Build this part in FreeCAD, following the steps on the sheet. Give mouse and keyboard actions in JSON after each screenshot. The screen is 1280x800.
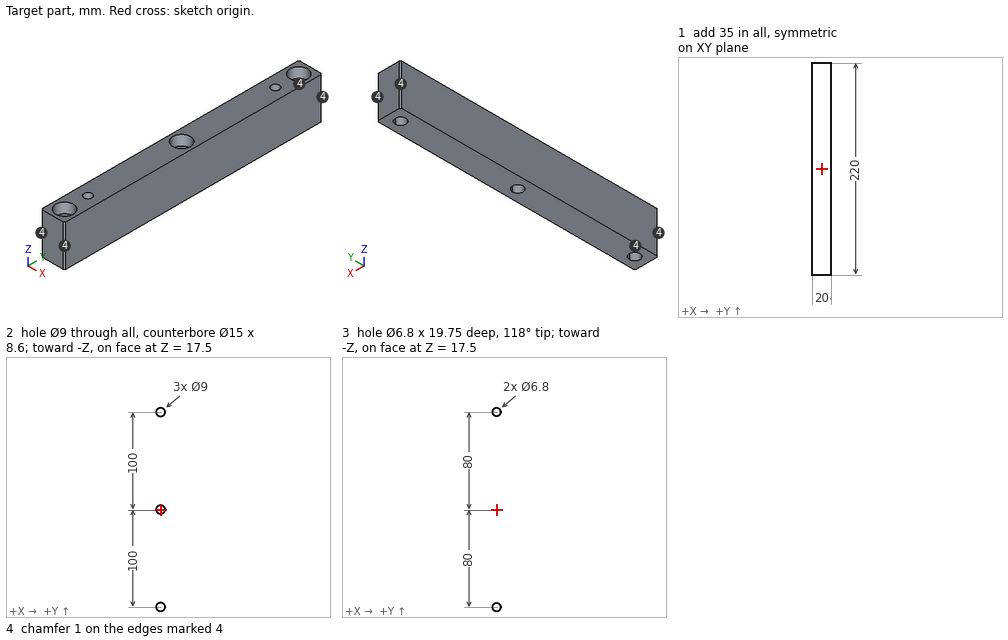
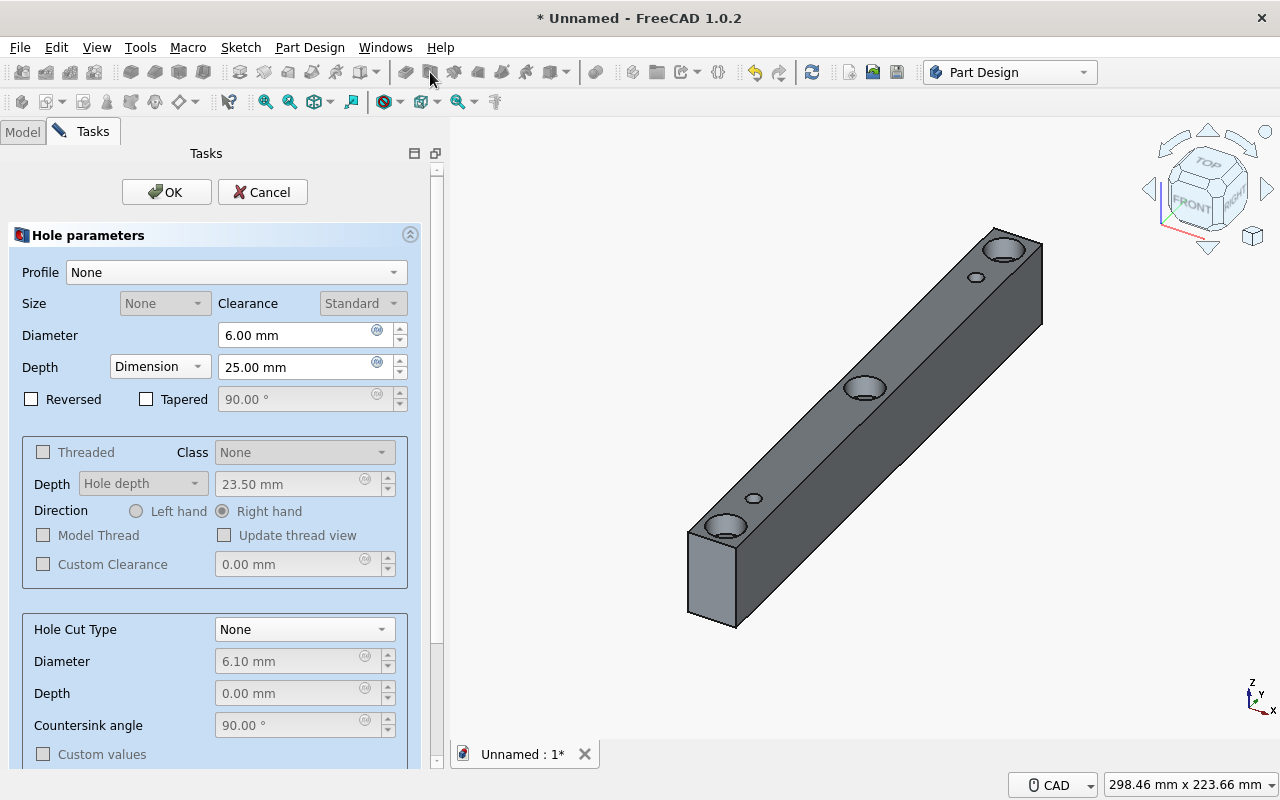
{"action": "triple_click", "coordinate": [305, 335]}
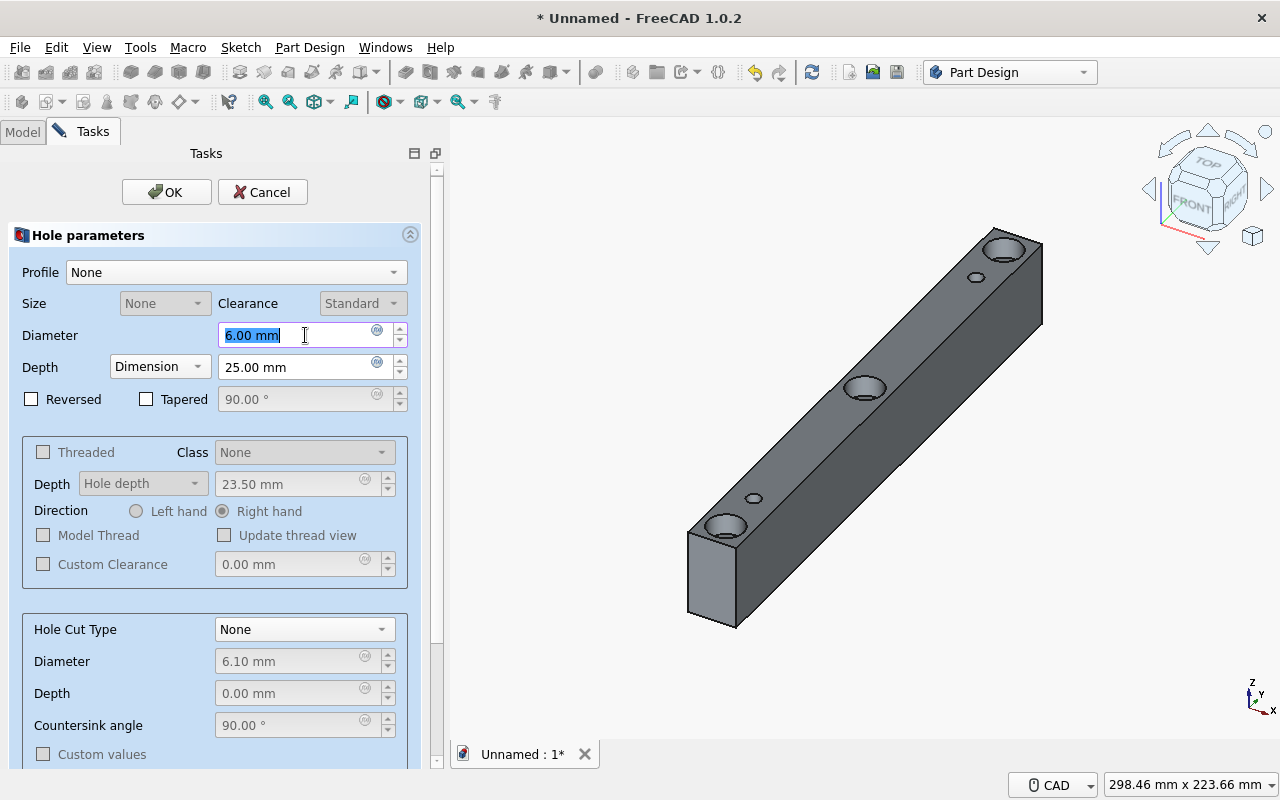
{"action": "type", "text": "6.8"}
{"action": "key", "text": "Tab"}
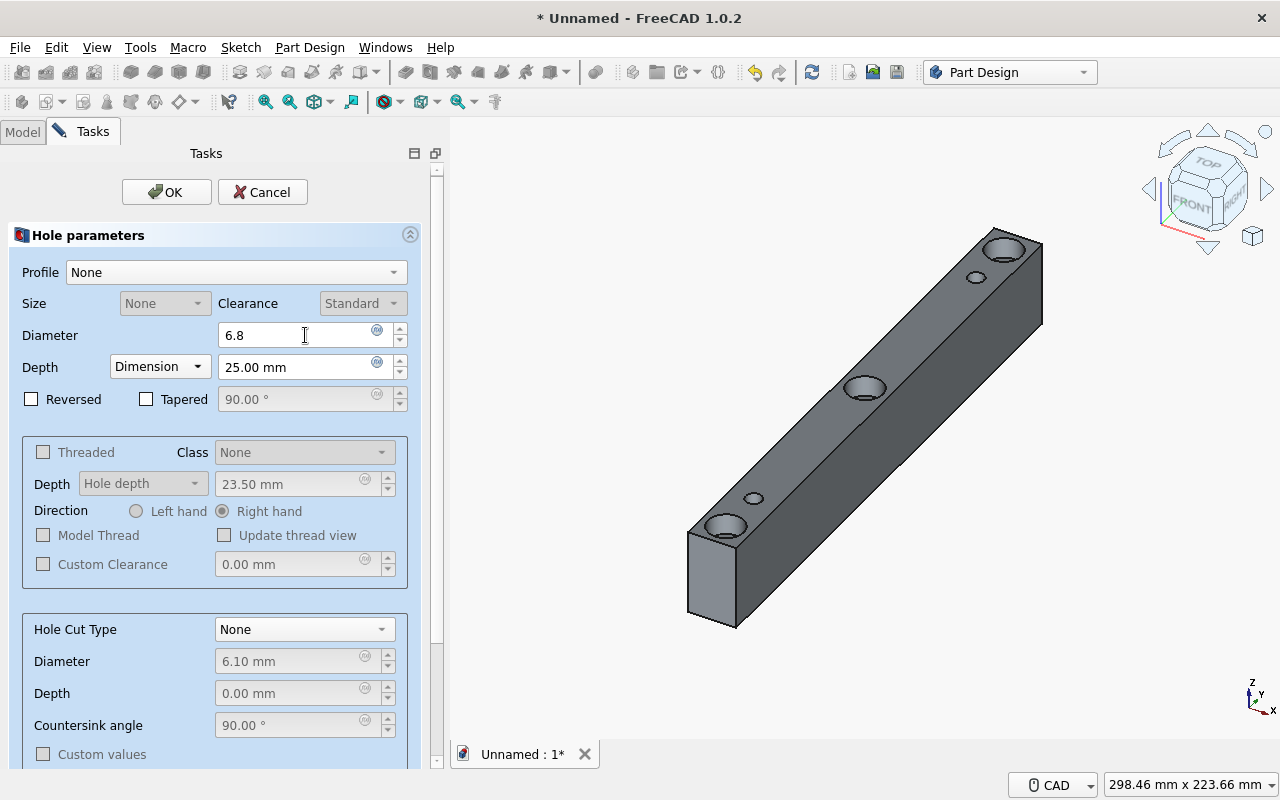
{"action": "triple_click", "coordinate": [305, 367]}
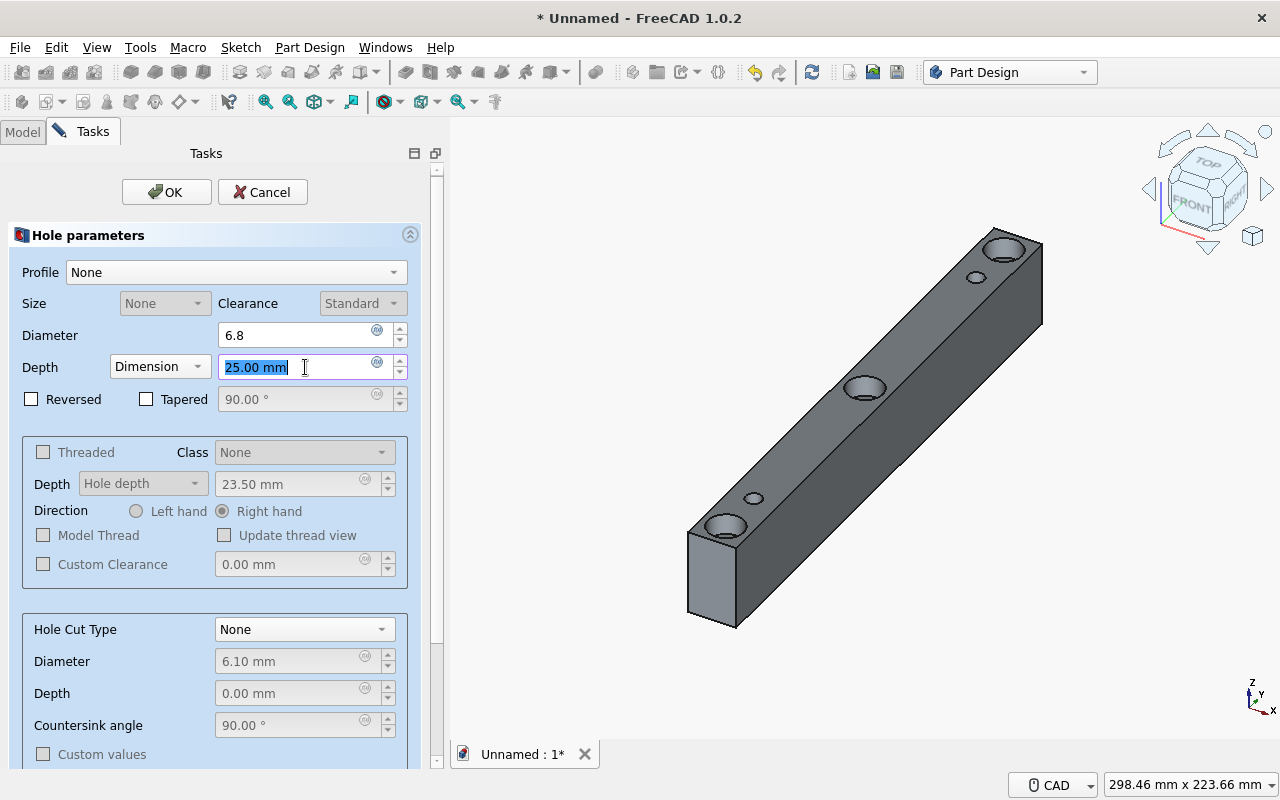
{"action": "type", "text": "19.75"}
{"action": "key", "text": "Tab"}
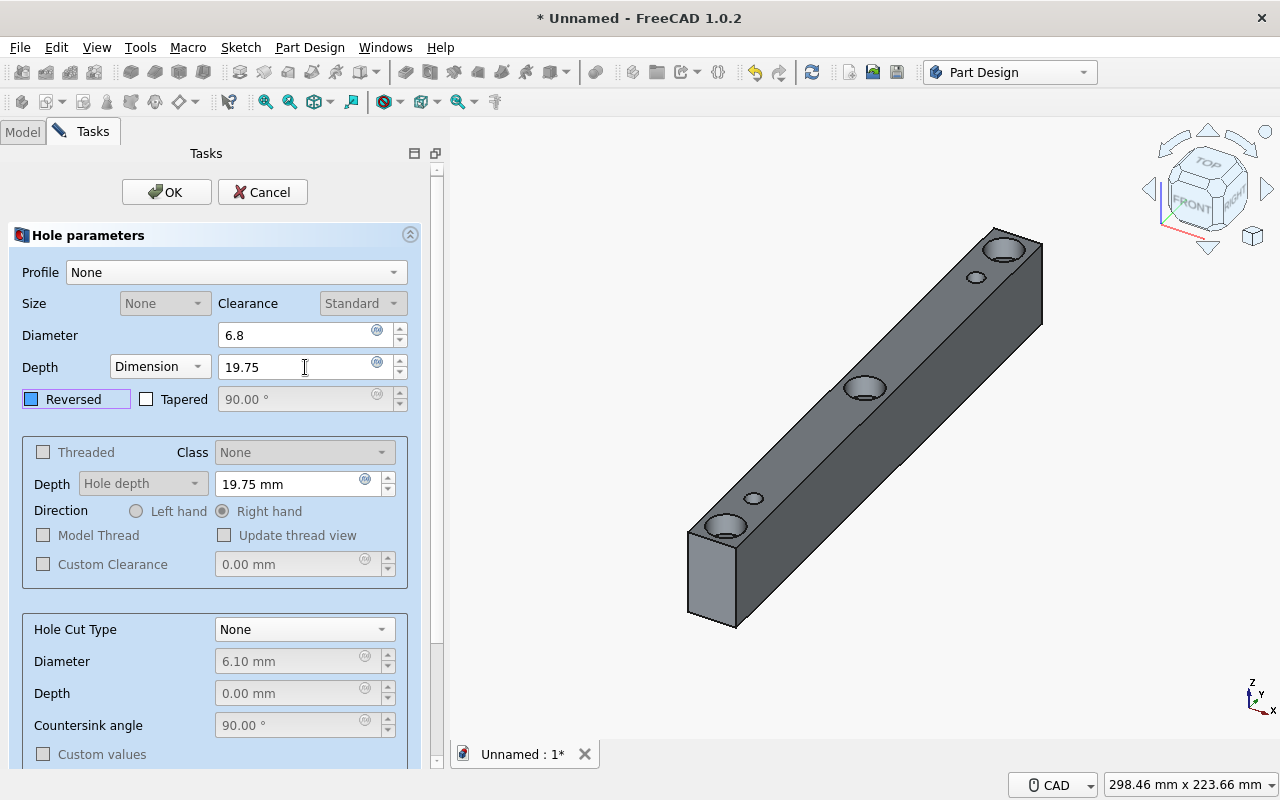
{"action": "left_click", "coordinate": [167, 192]}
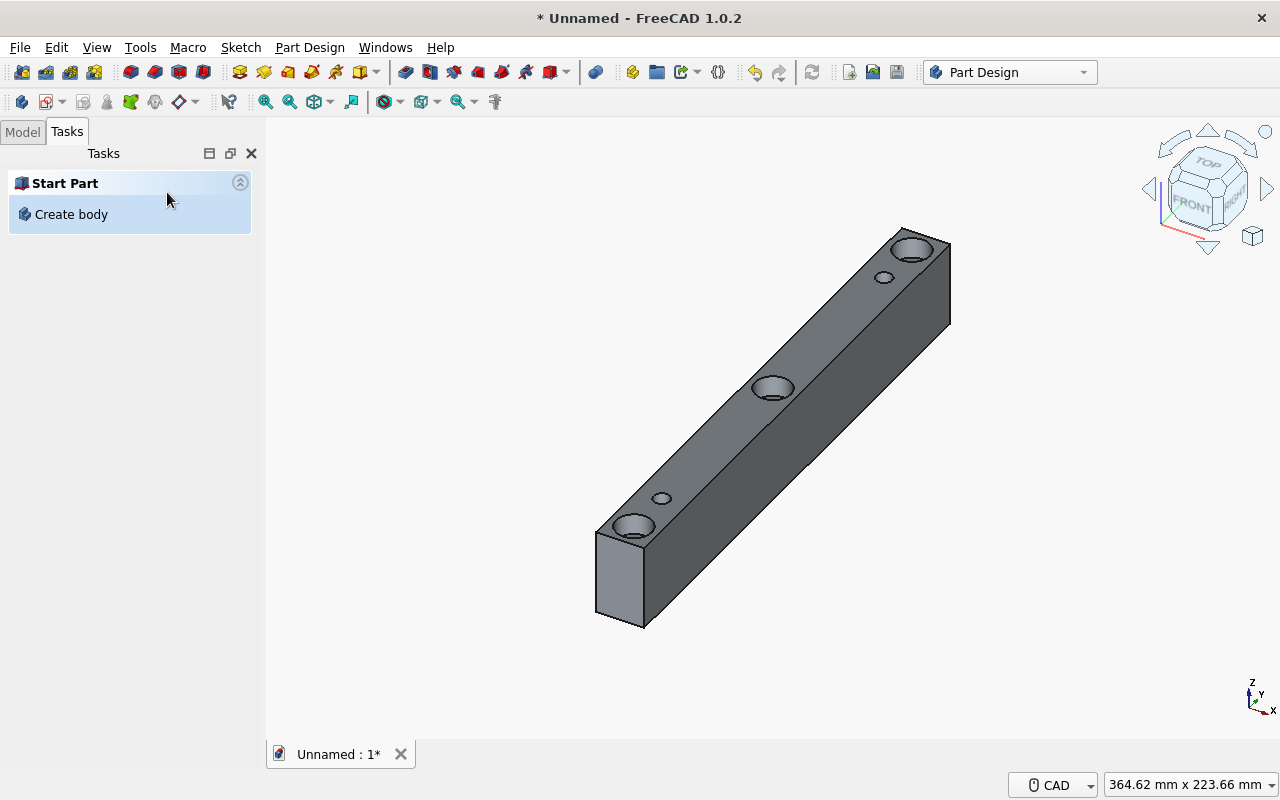
{"action": "left_click", "coordinate": [644, 587]}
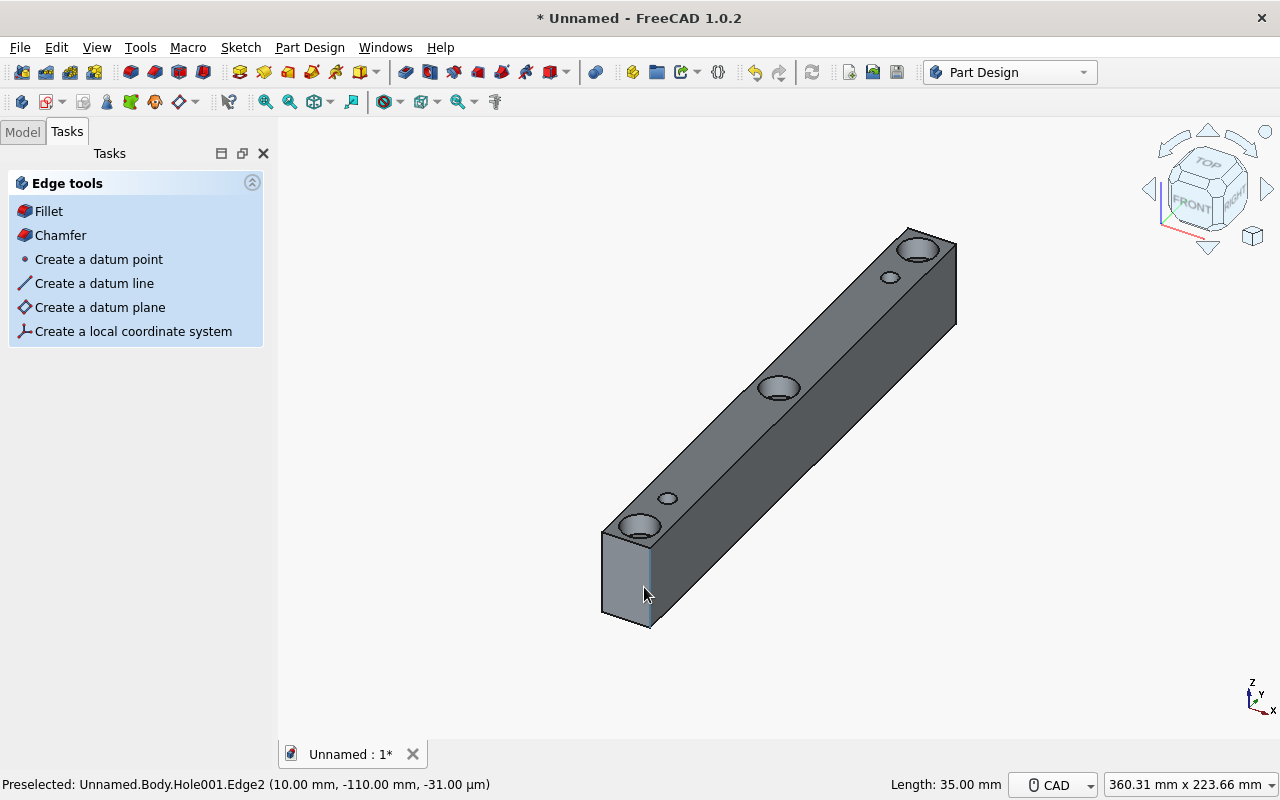
{"action": "key", "text": "0"}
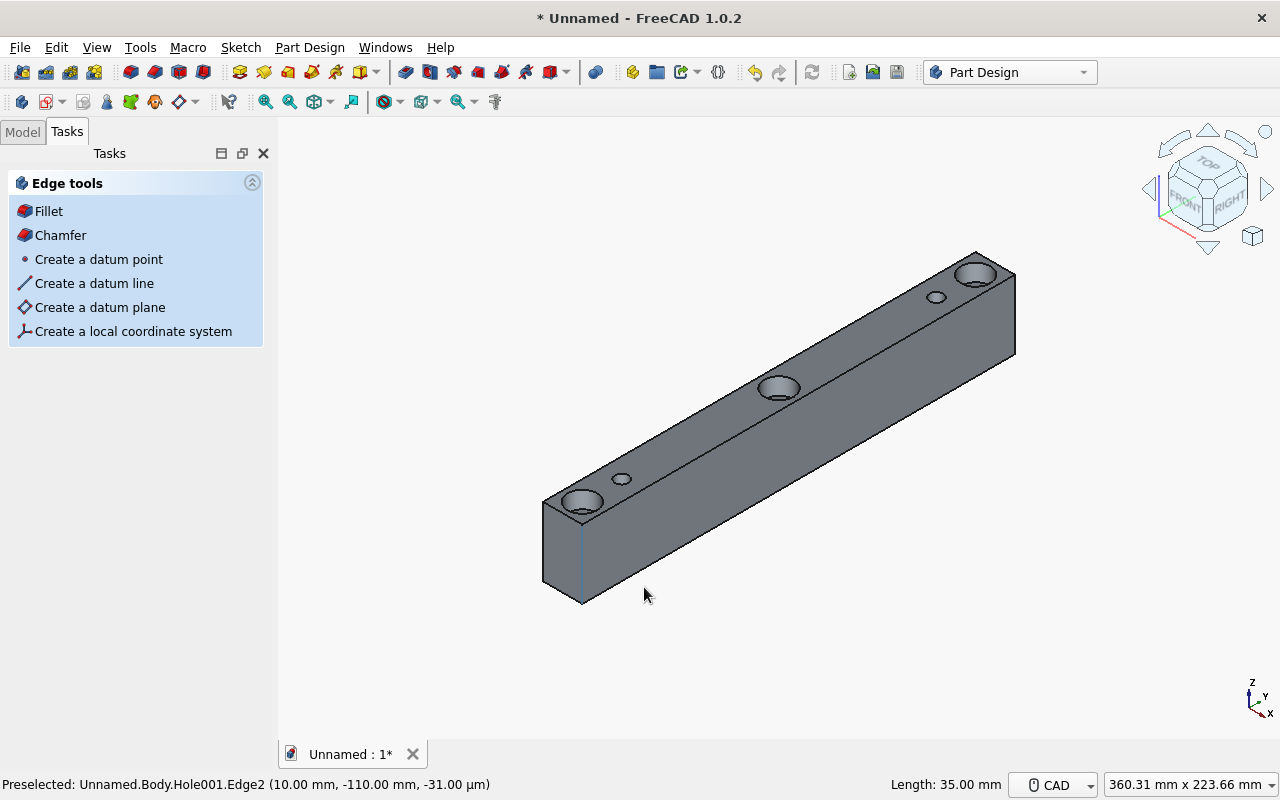
{"action": "key", "text": "2"}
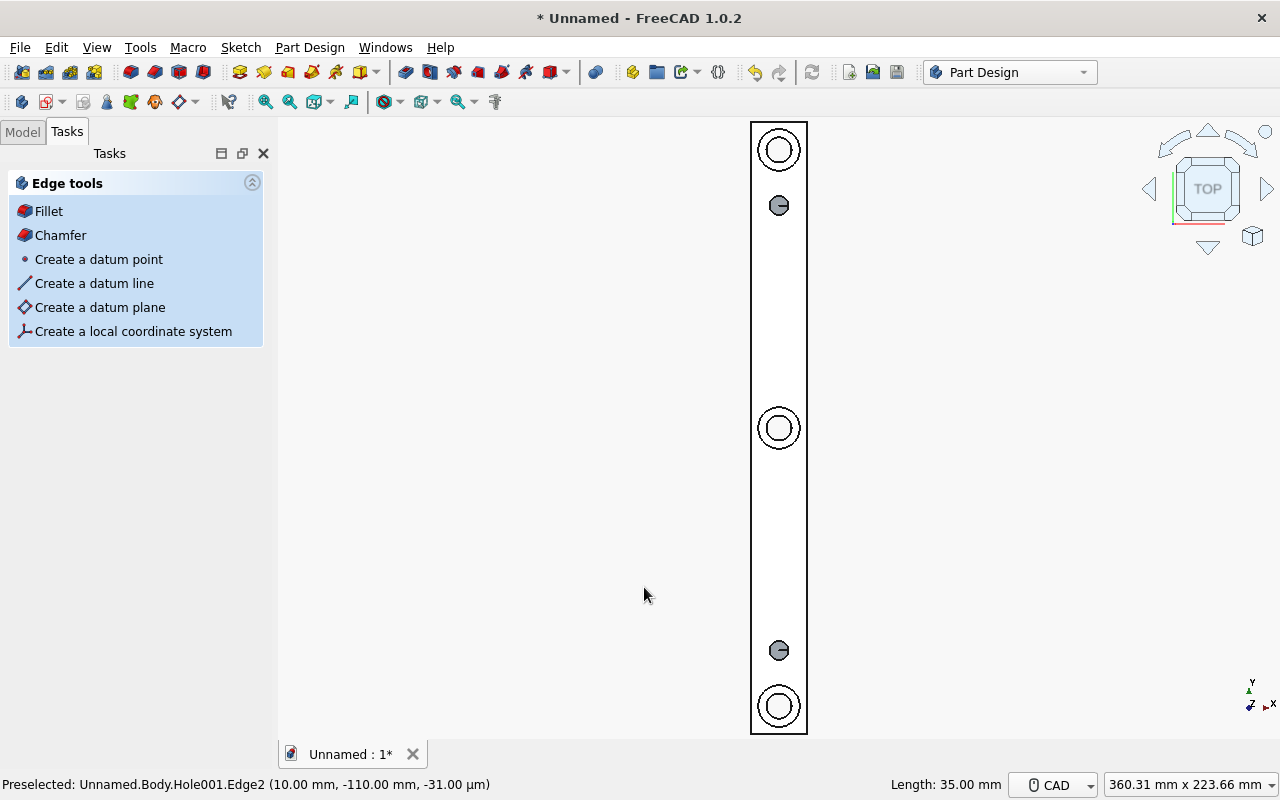
{"action": "key", "text": "1"}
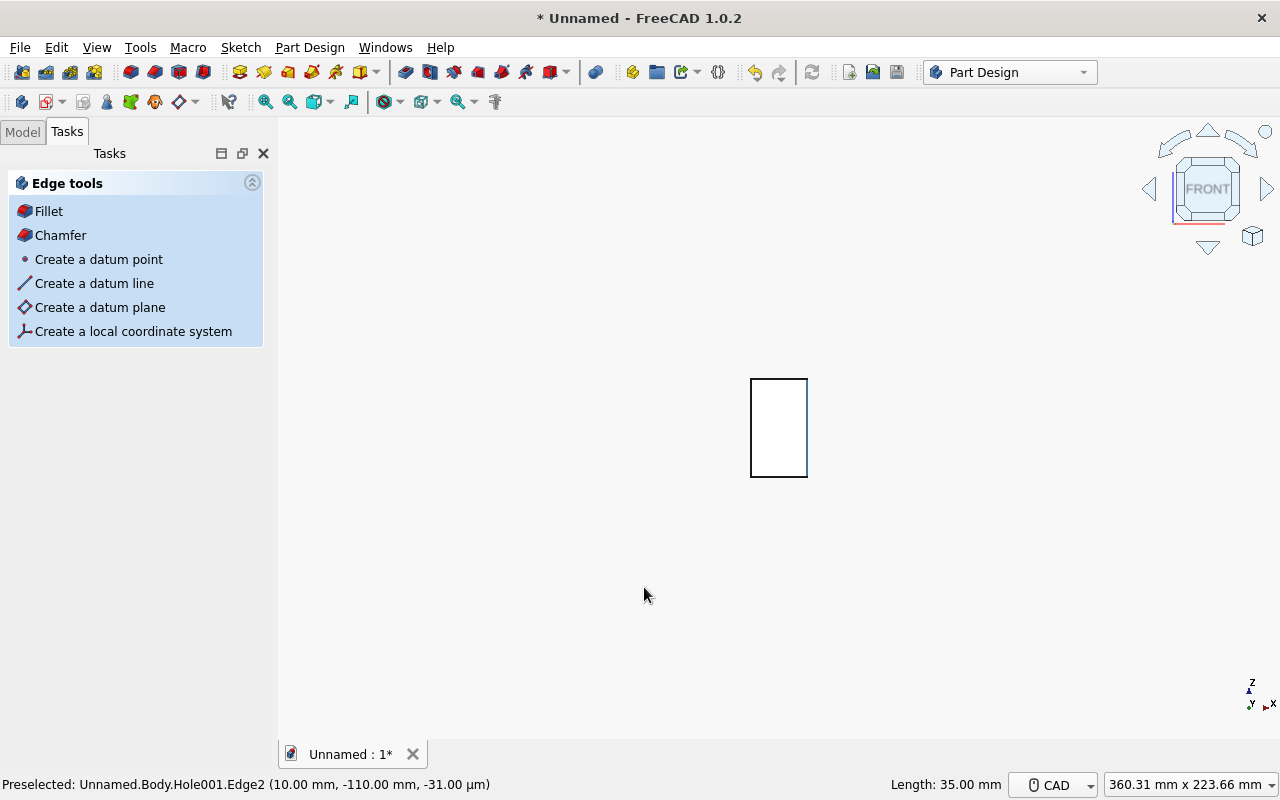
{"action": "left_click", "coordinate": [266, 102]}